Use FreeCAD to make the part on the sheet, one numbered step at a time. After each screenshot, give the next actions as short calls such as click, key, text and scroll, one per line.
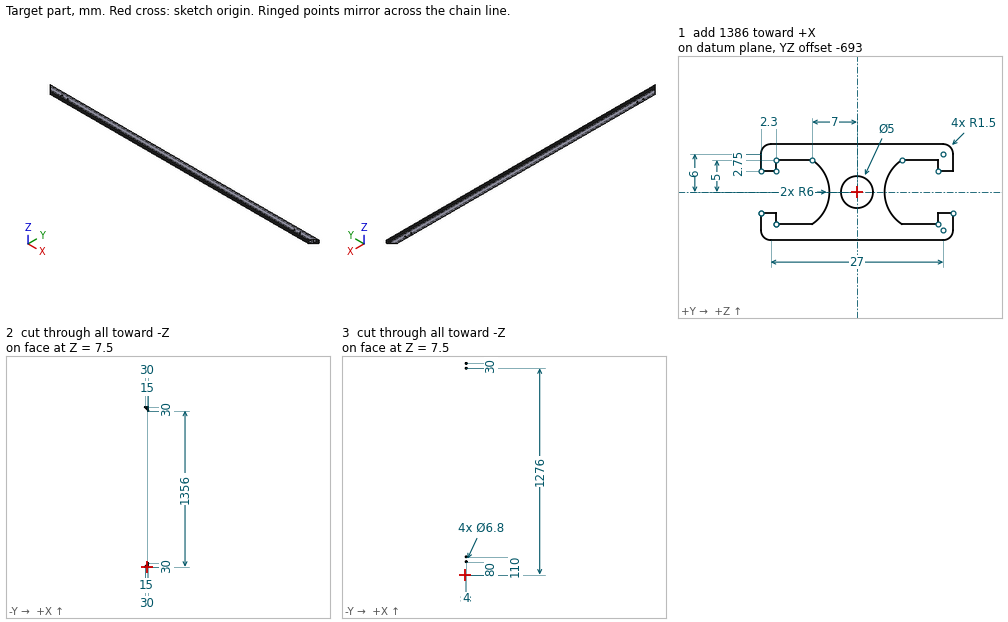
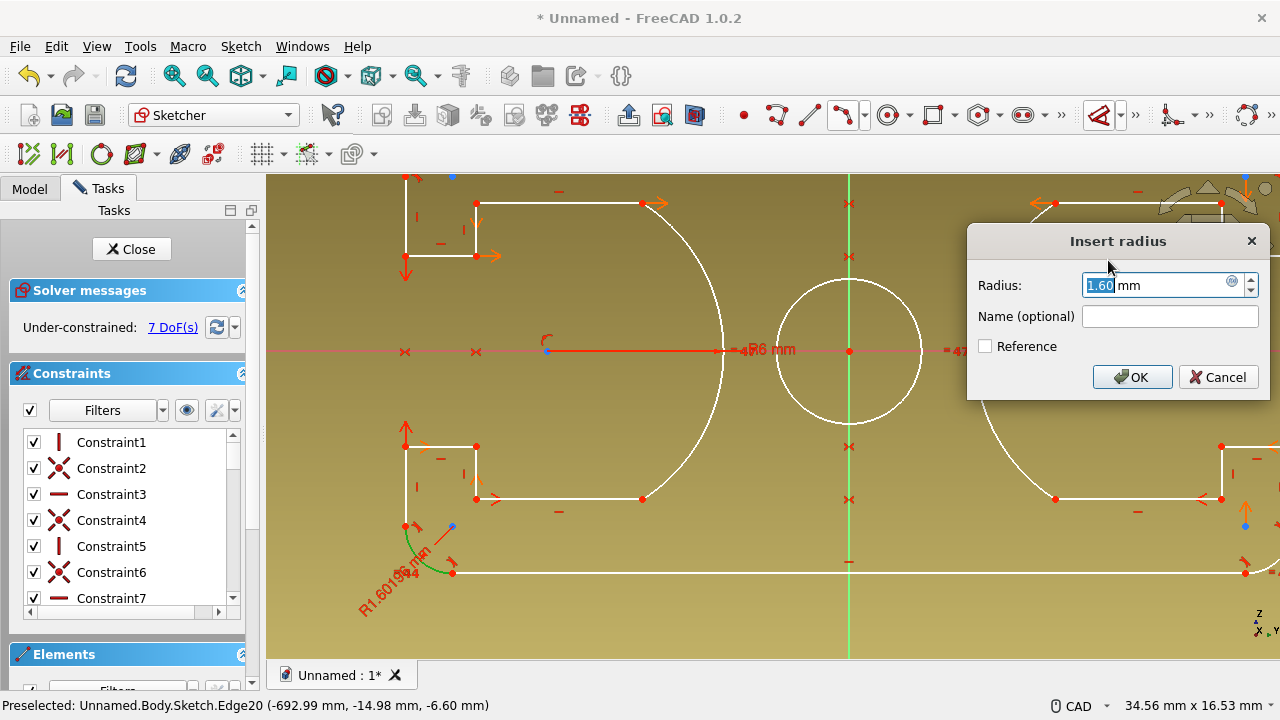
text(1.5)
key(Return)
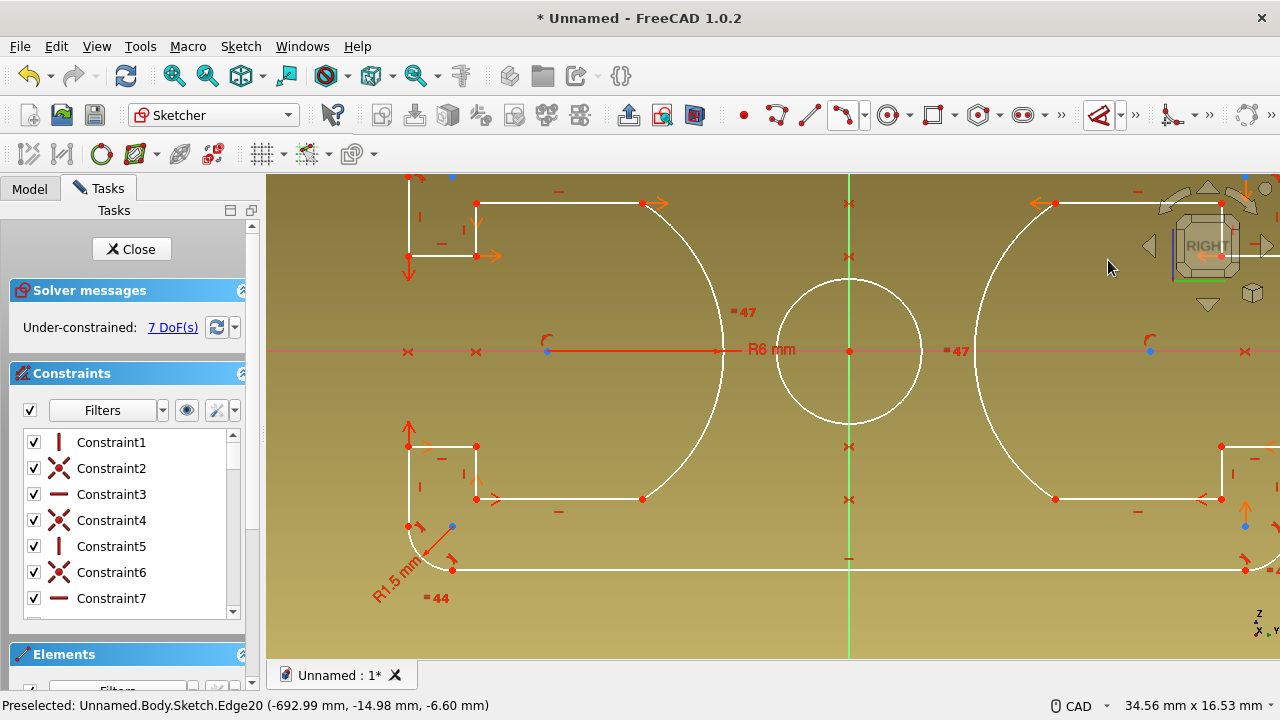
click(900, 300)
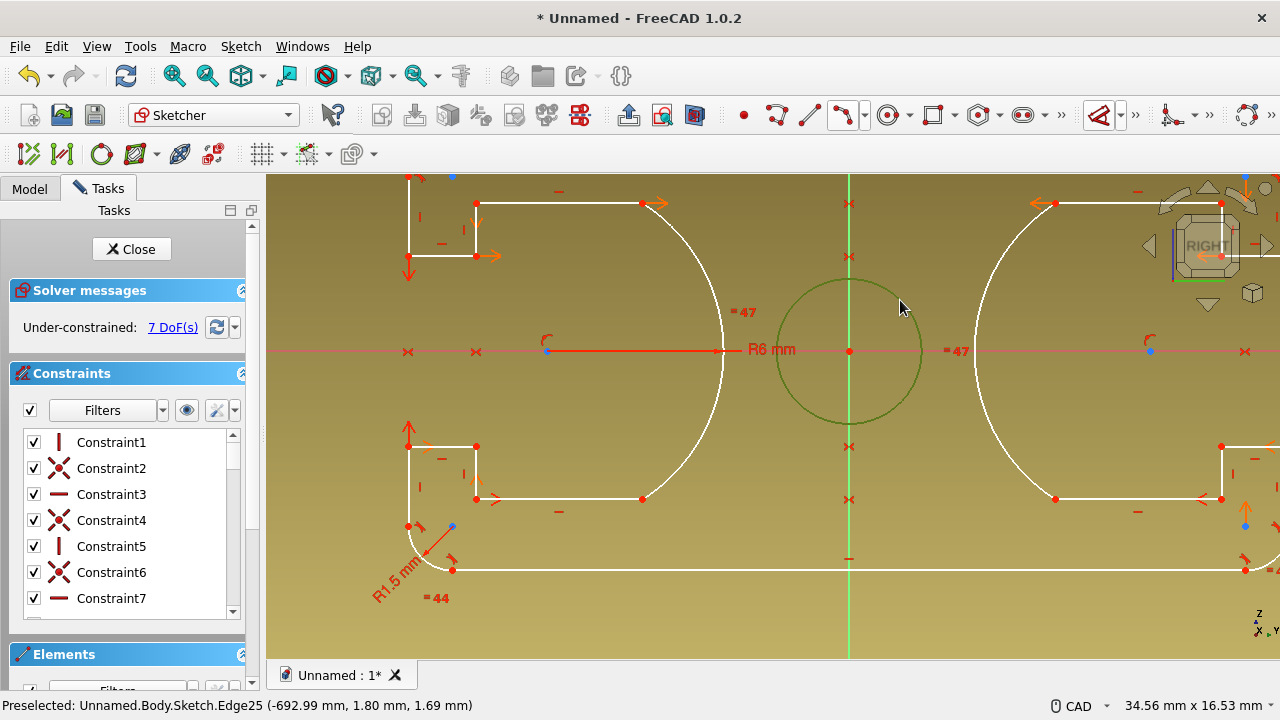
click(1120, 116)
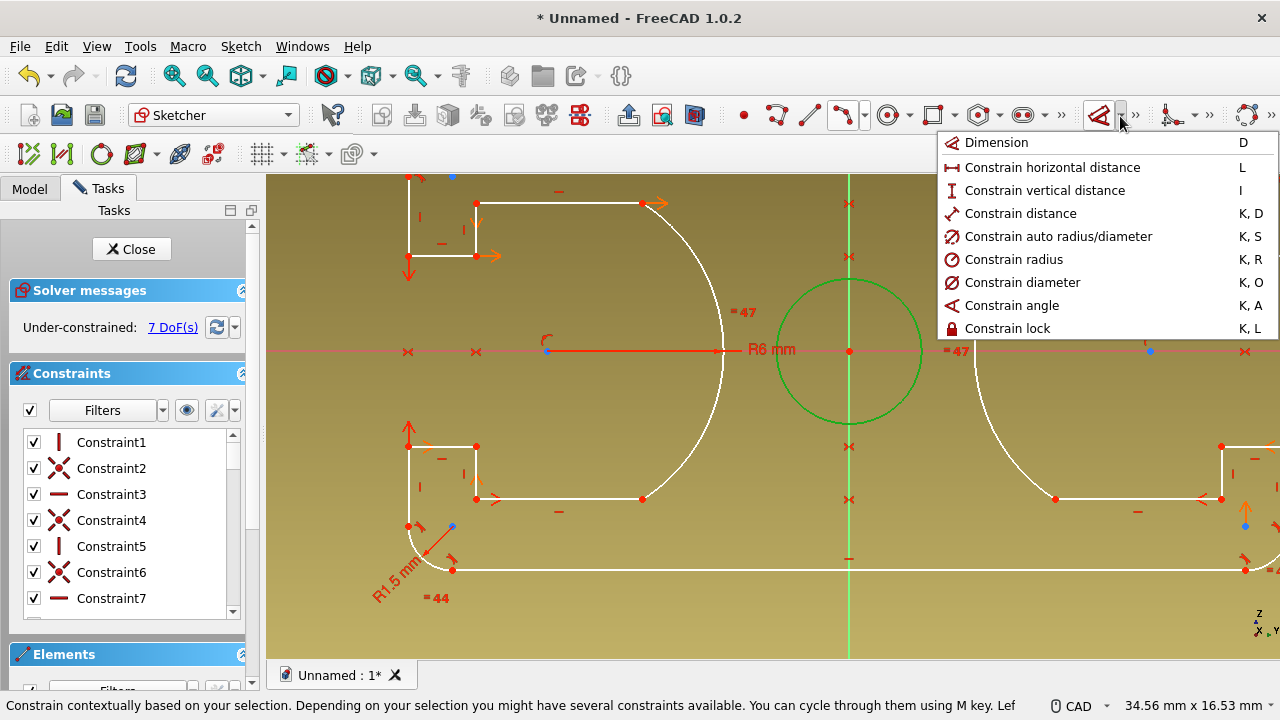
click(1108, 282)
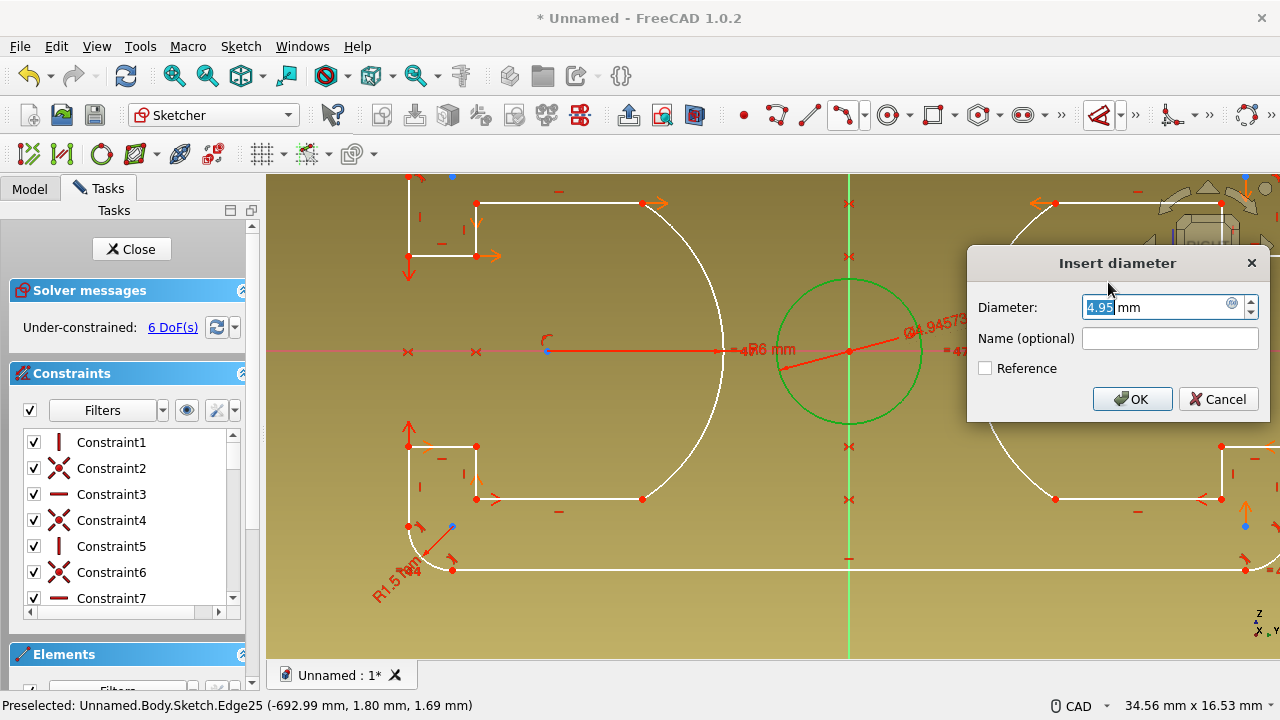
text(5)
key(Return)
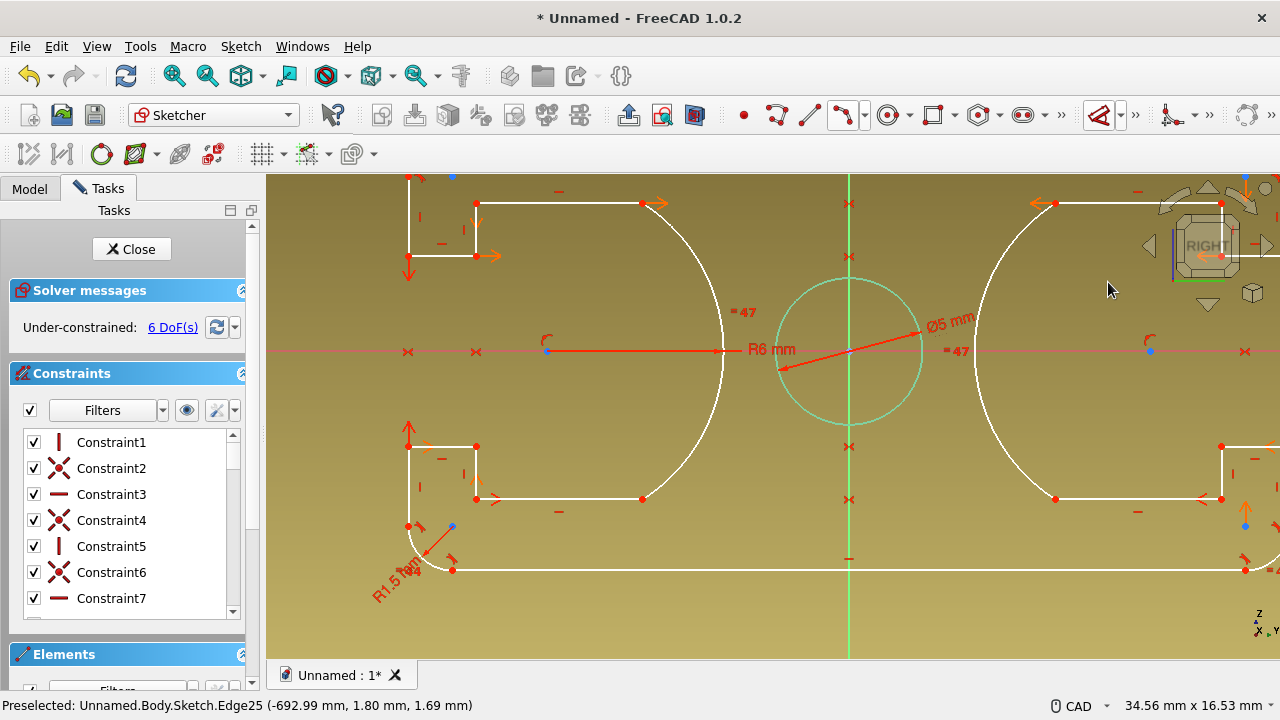
click(691, 570)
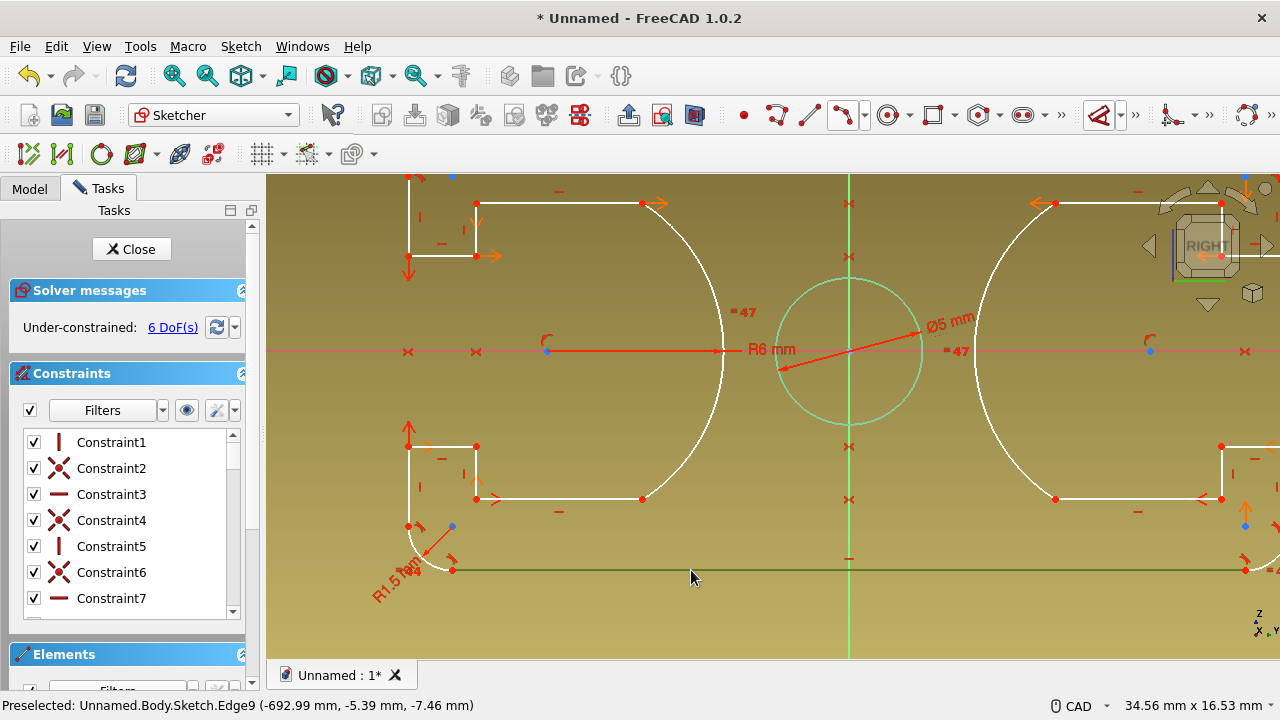
key(l)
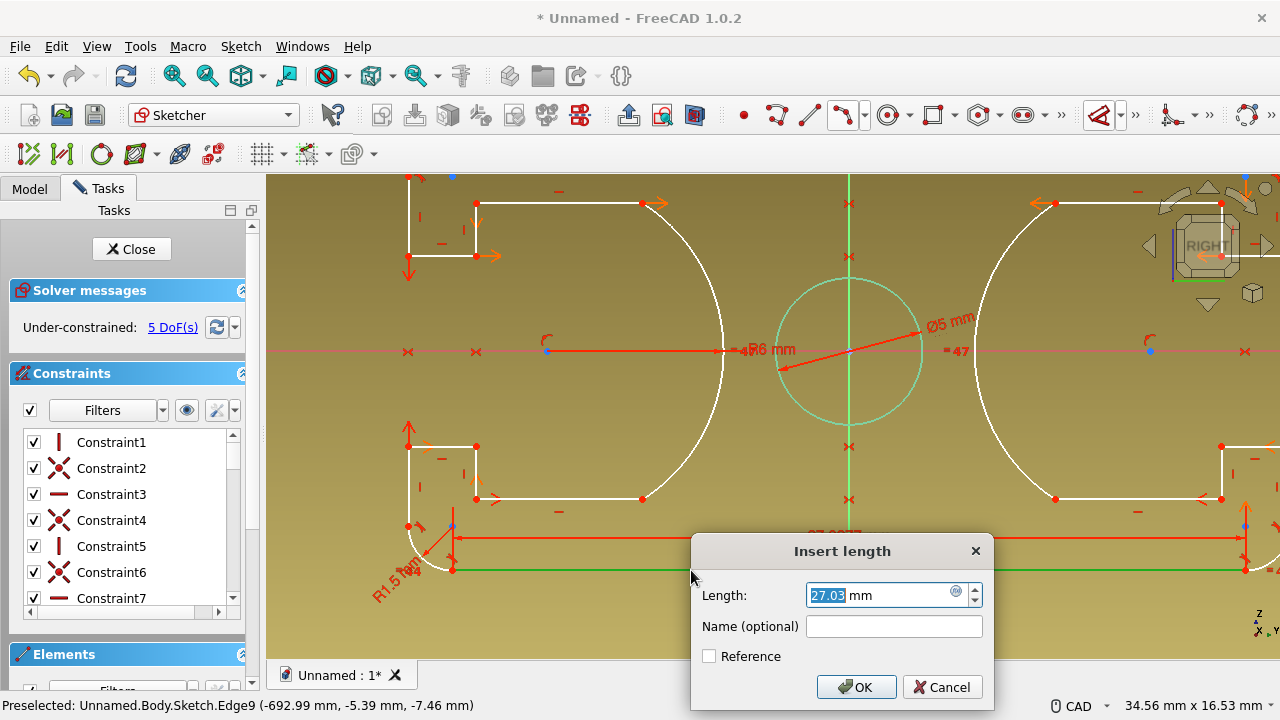
text(27)
key(Return)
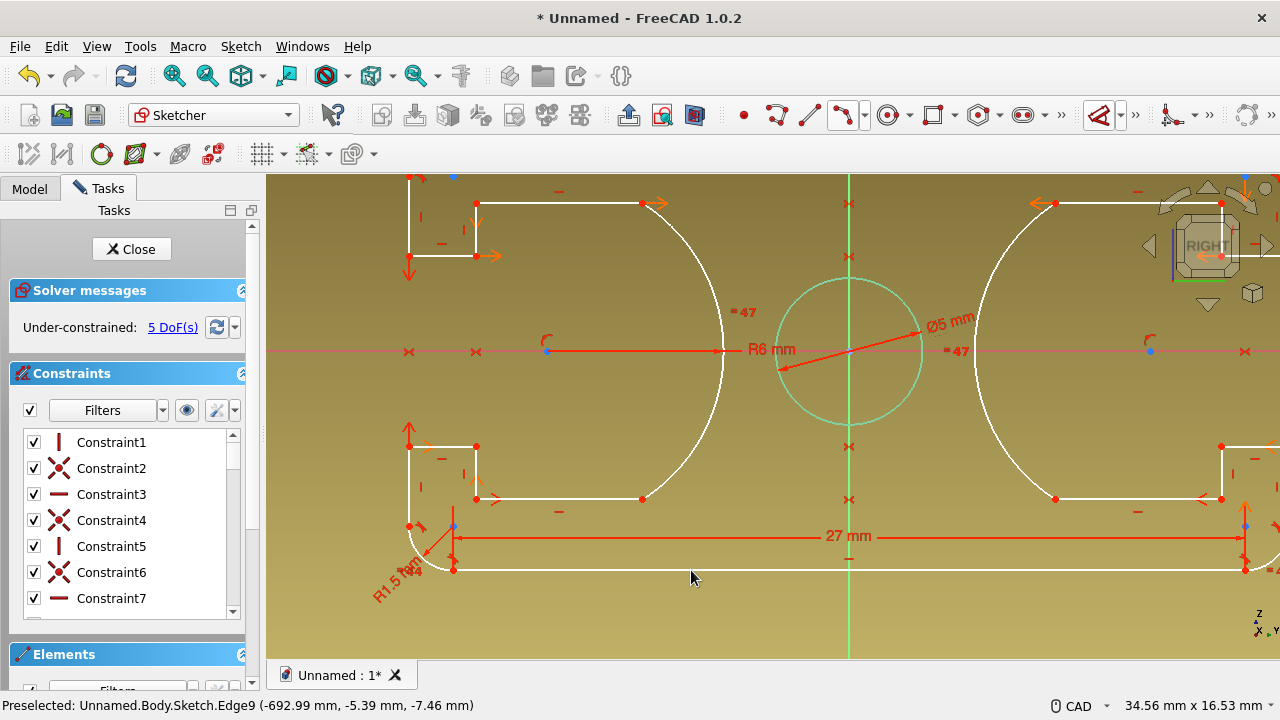
scroll(410, 549, down, 2)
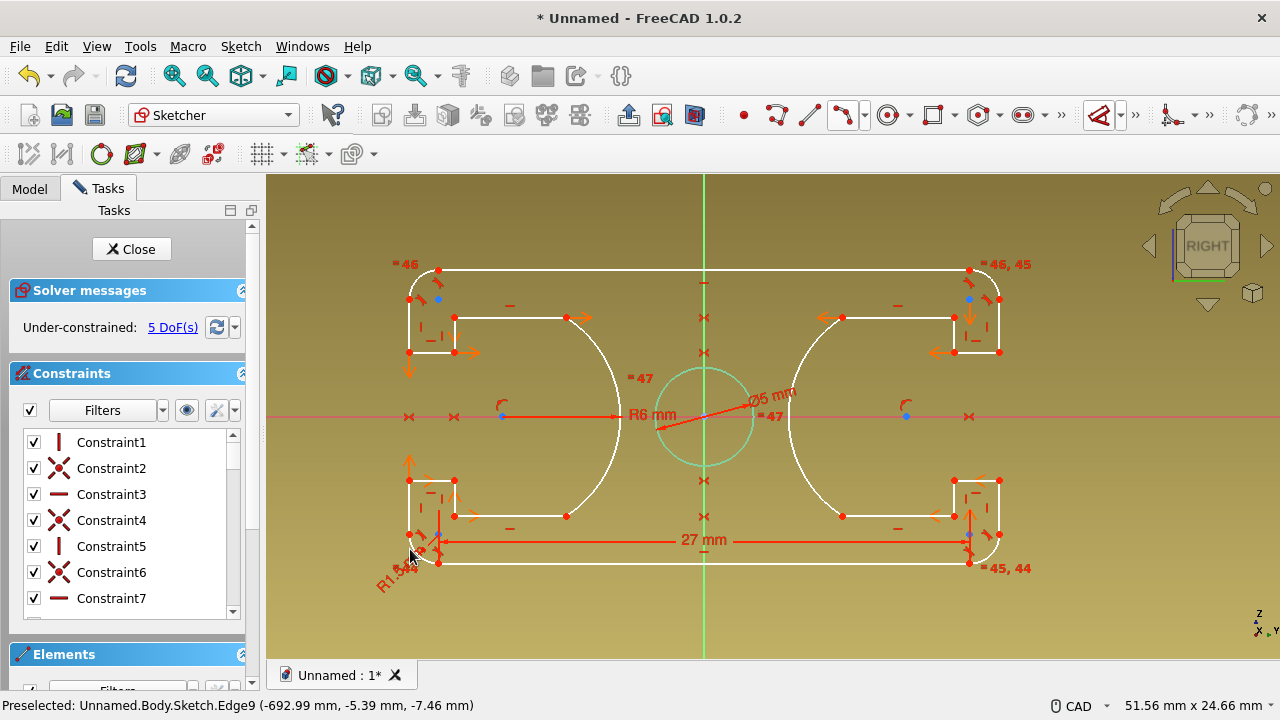
click(409, 300)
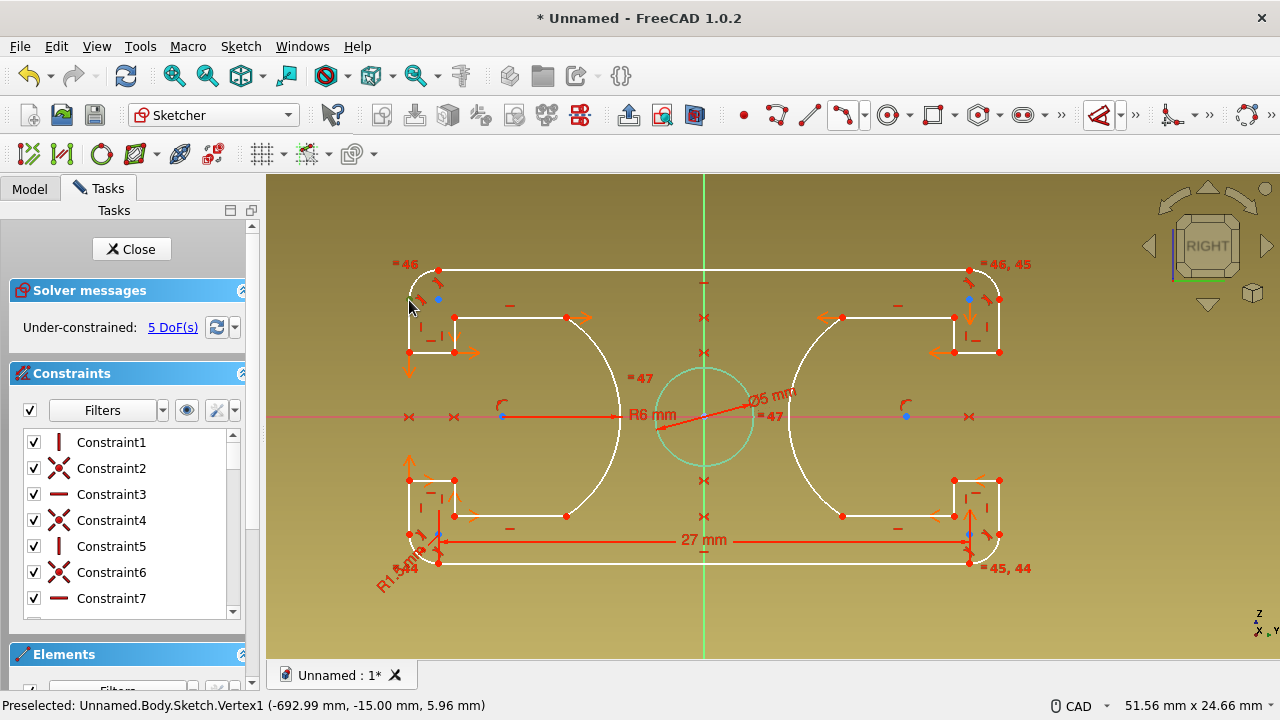
key(i)